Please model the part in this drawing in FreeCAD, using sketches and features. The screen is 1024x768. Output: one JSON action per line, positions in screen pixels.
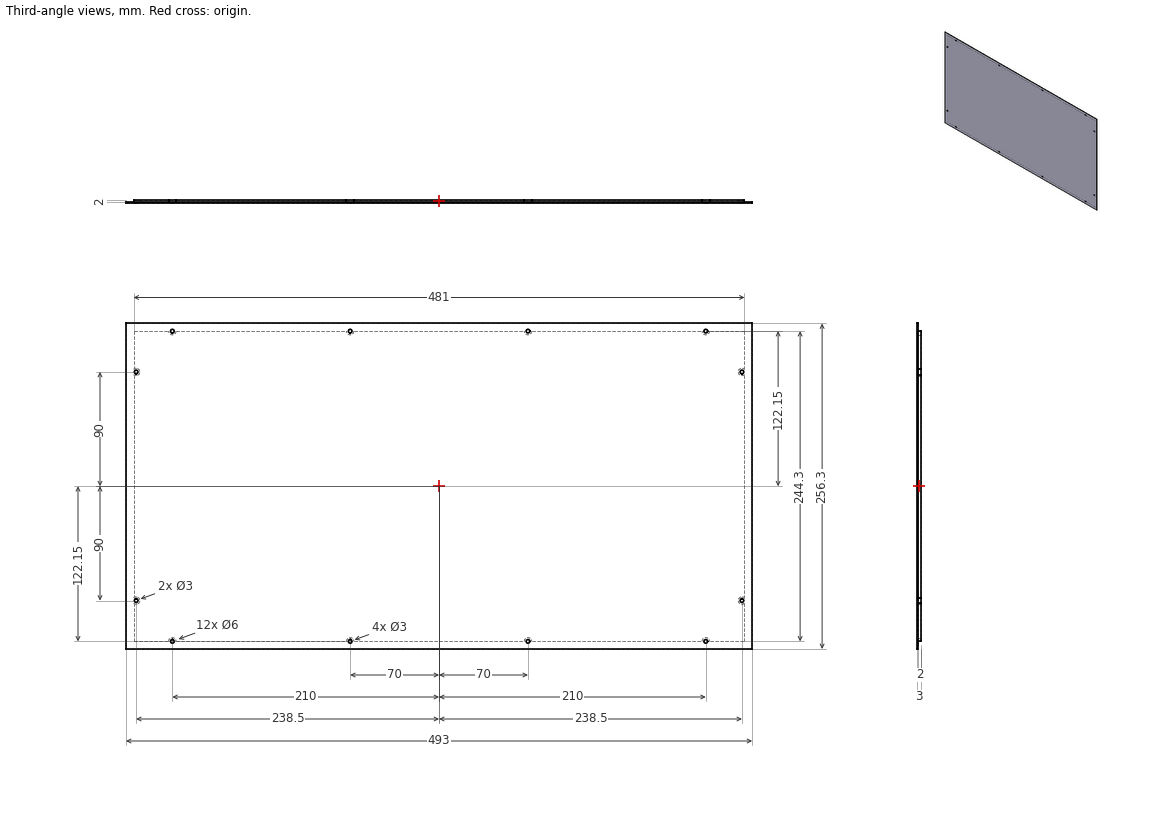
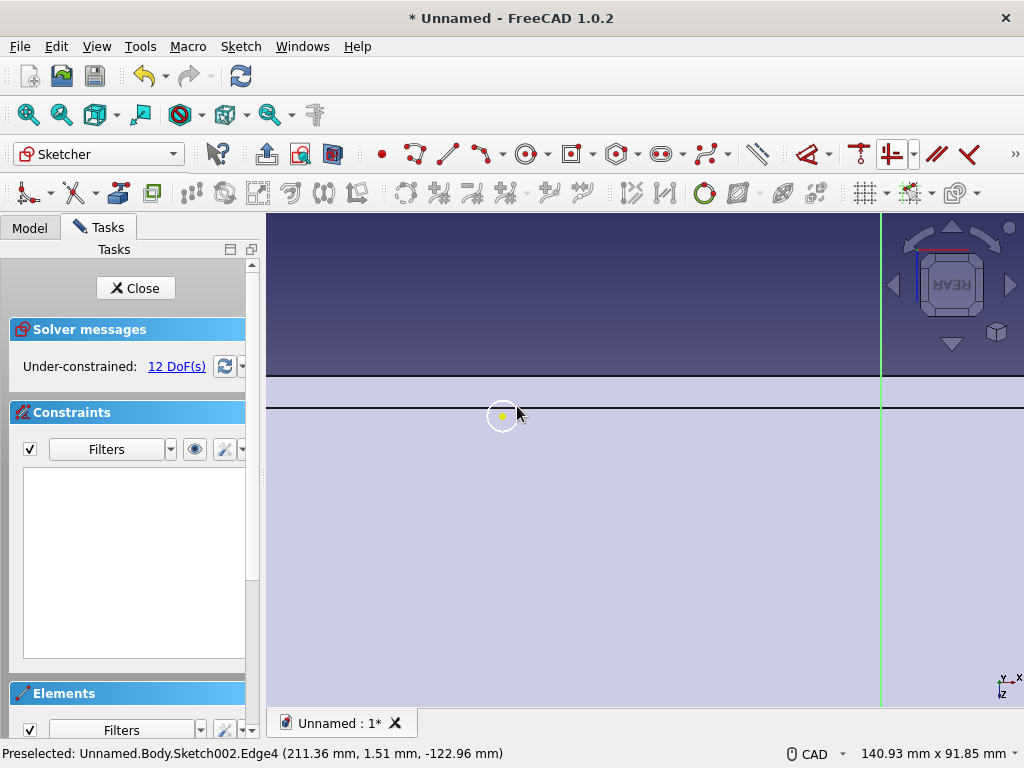
{"action": "left_click", "coordinate": [514, 405]}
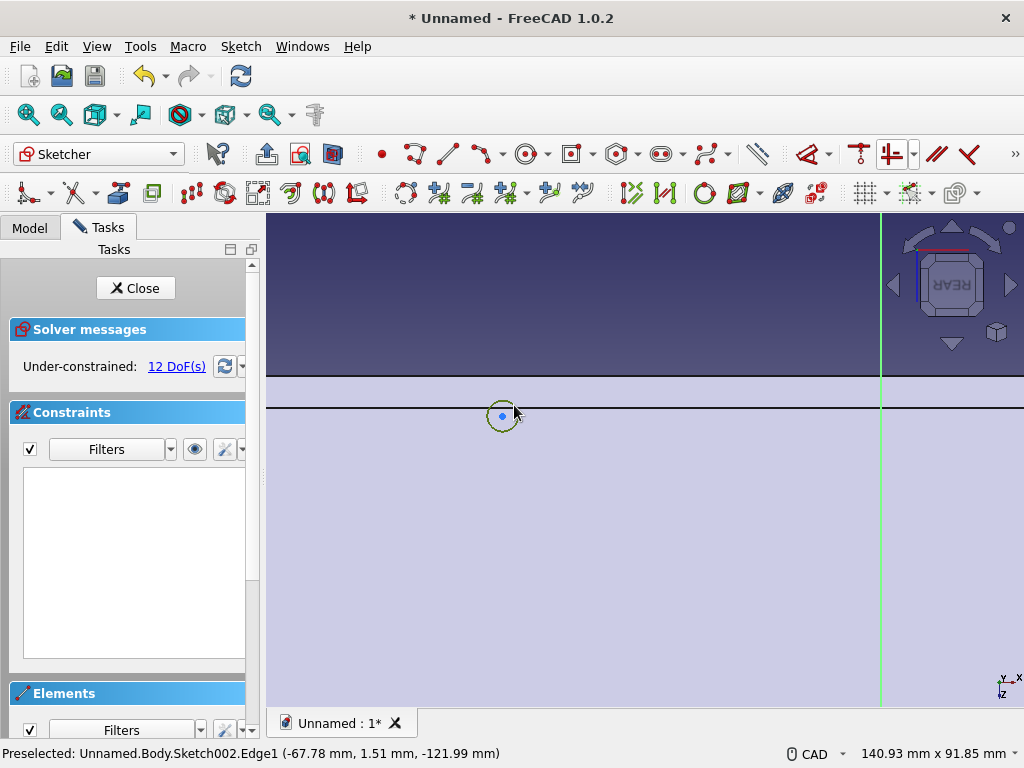
{"action": "scroll", "coordinate": [516, 406], "scroll_direction": "down", "scroll_amount": 9}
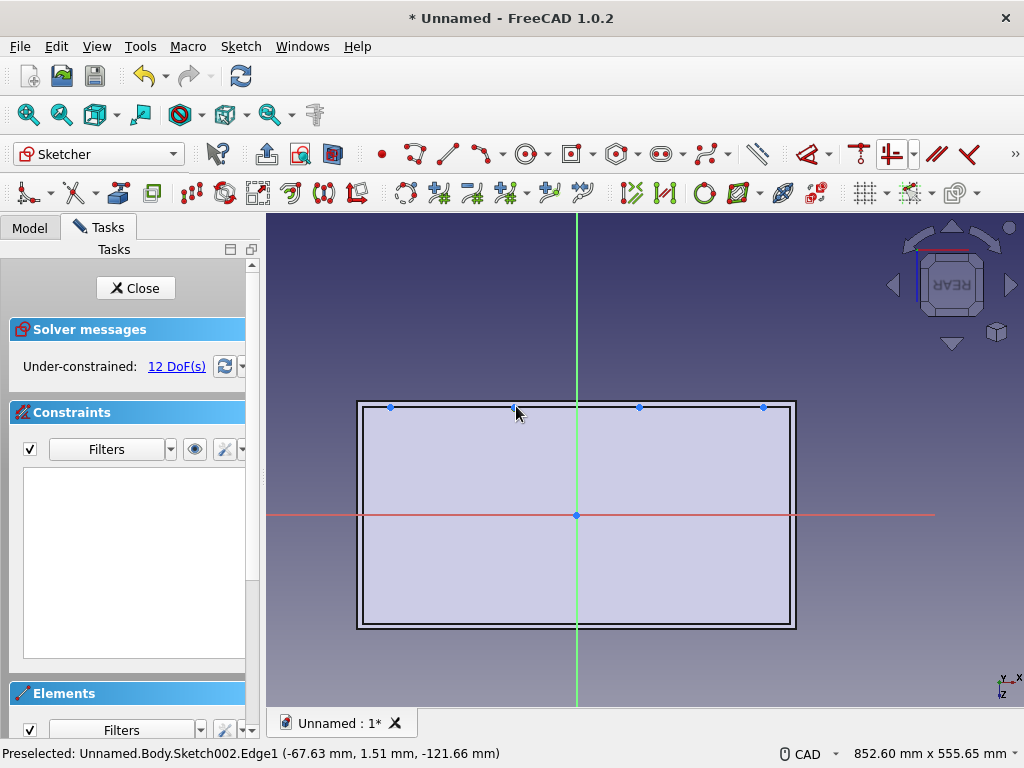
{"action": "scroll", "coordinate": [392, 406], "scroll_direction": "up", "scroll_amount": 9}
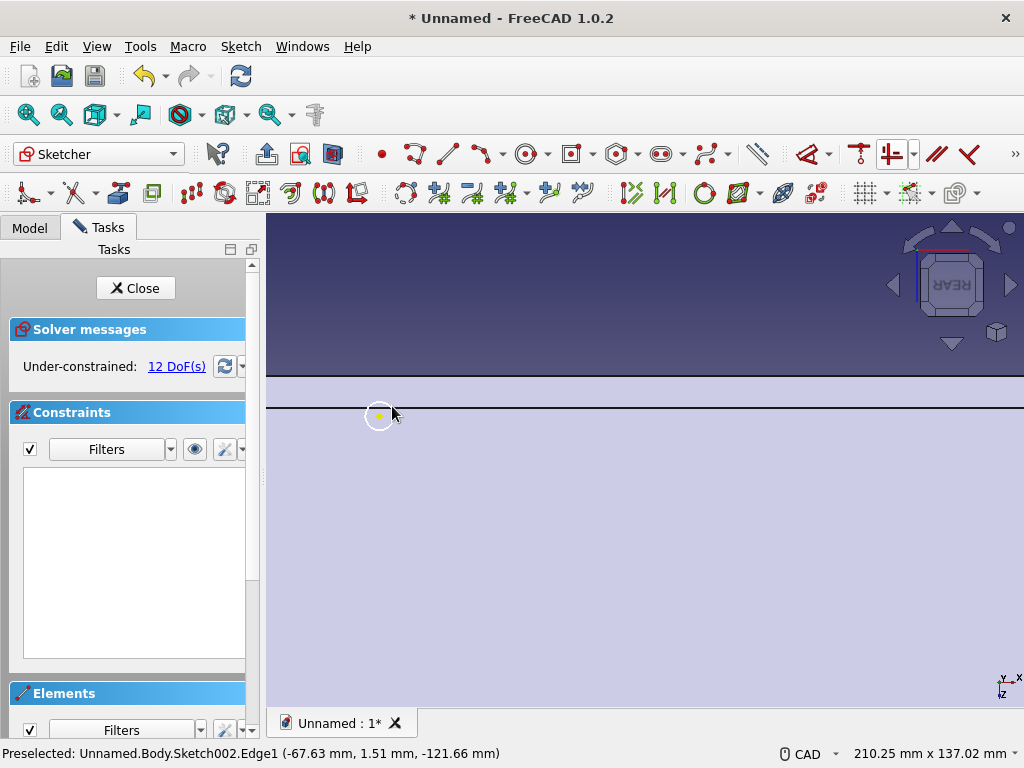
{"action": "left_click", "coordinate": [390, 406]}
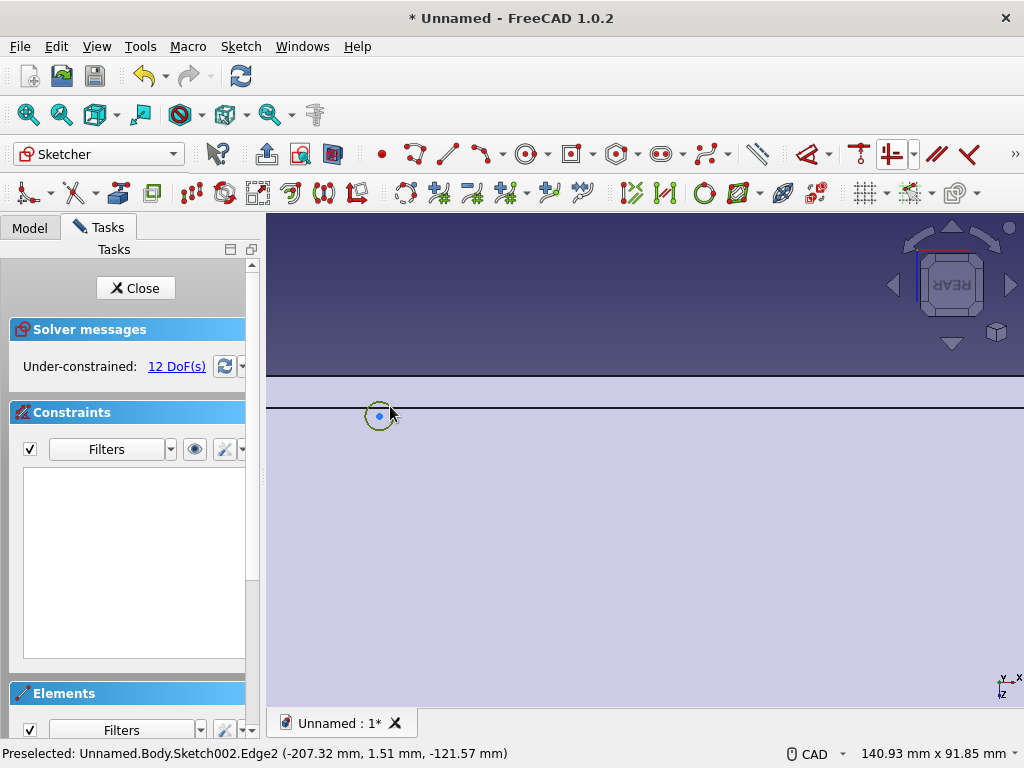
{"action": "scroll", "coordinate": [392, 406], "scroll_direction": "down", "scroll_amount": 9}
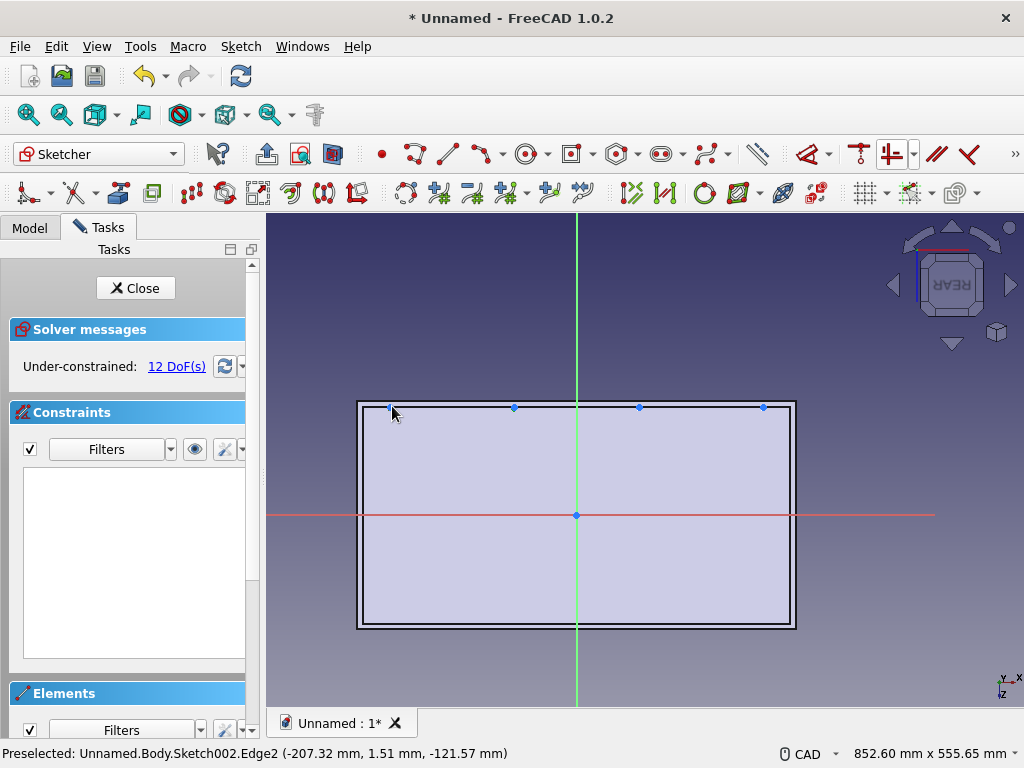
{"action": "scroll", "coordinate": [641, 406], "scroll_direction": "up", "scroll_amount": 9}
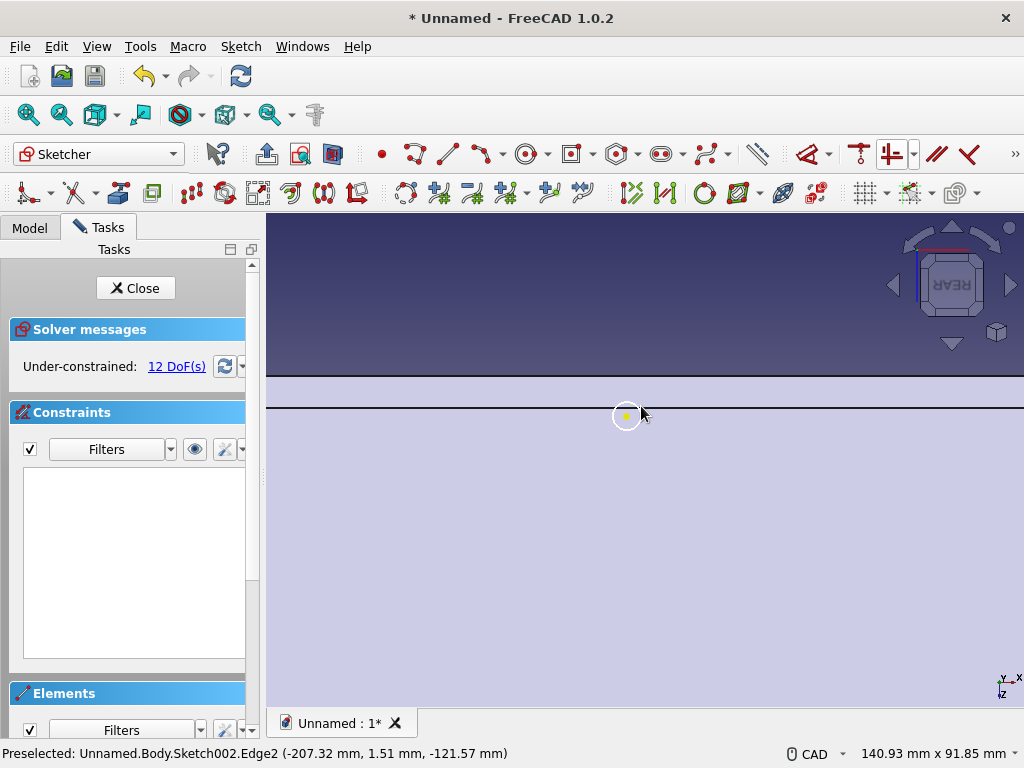
{"action": "left_click", "coordinate": [637, 406]}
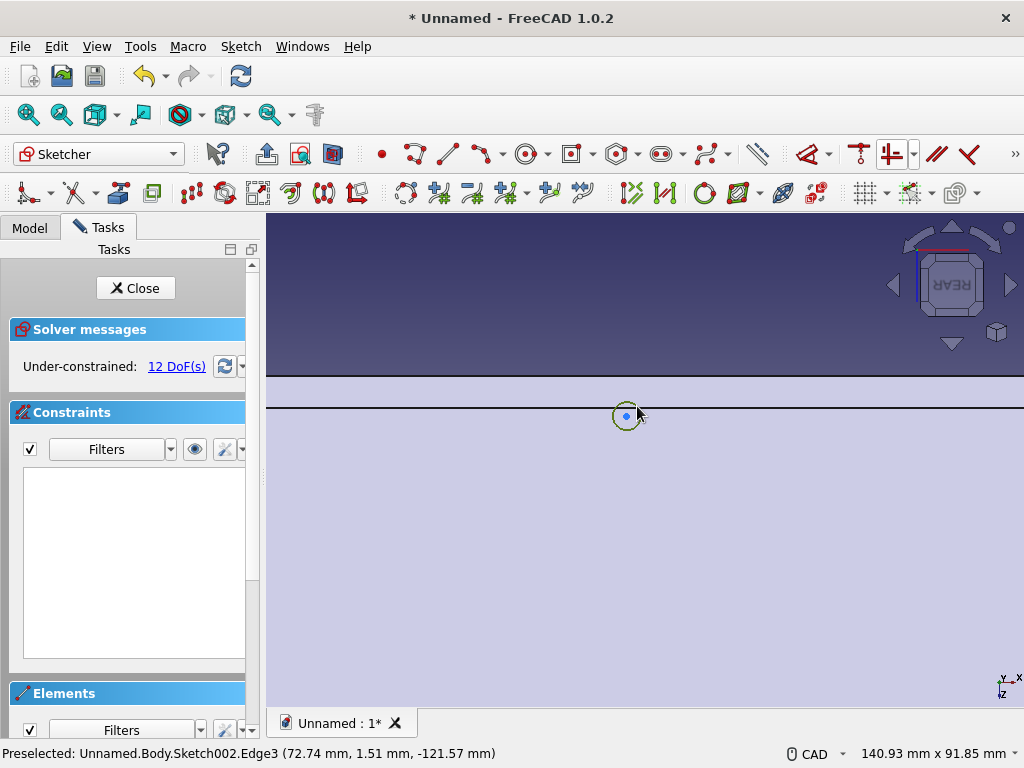
{"action": "scroll", "coordinate": [641, 406], "scroll_direction": "down", "scroll_amount": 9}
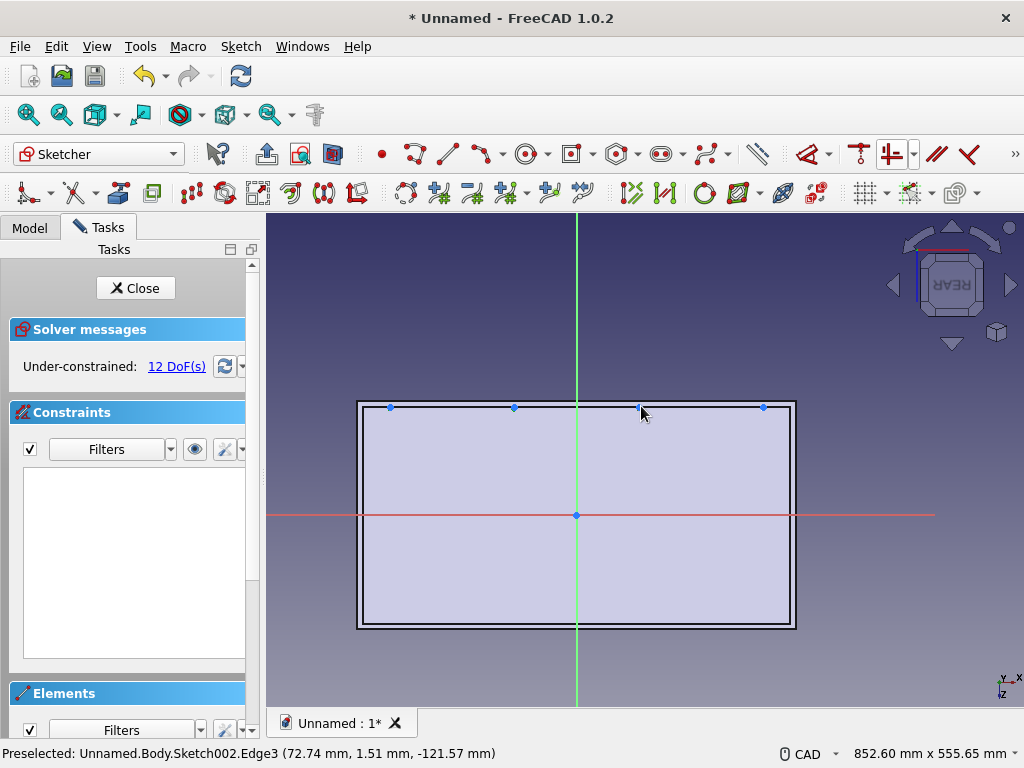
{"action": "scroll", "coordinate": [765, 406], "scroll_direction": "up", "scroll_amount": 9}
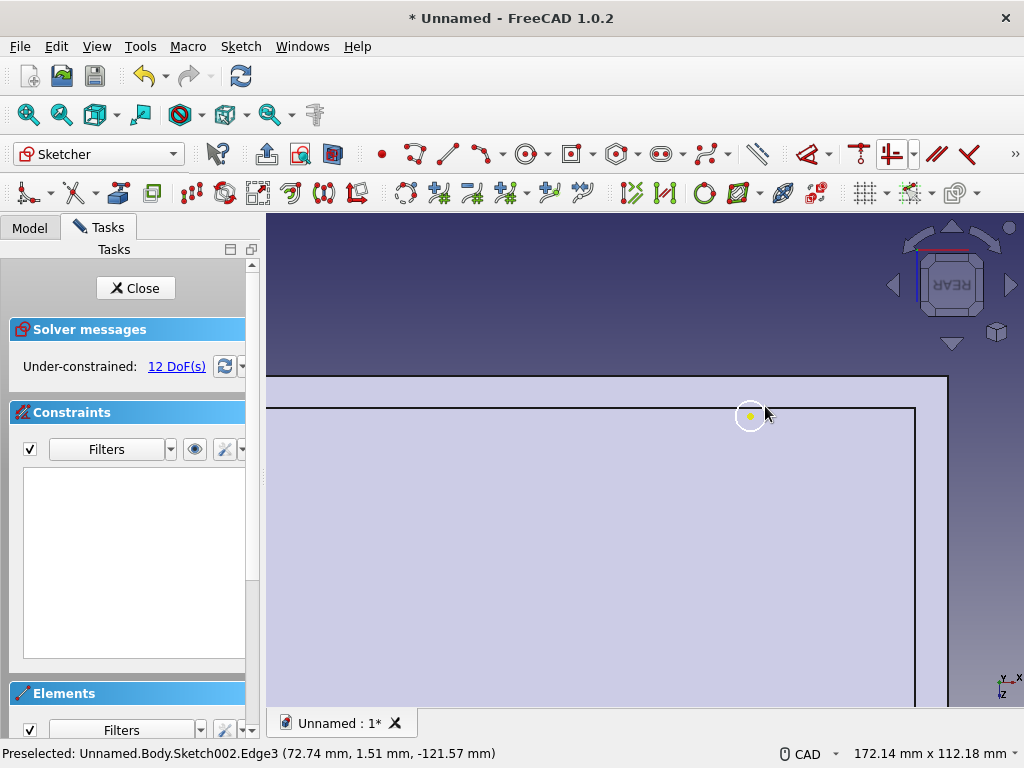
{"action": "left_click", "coordinate": [761, 405]}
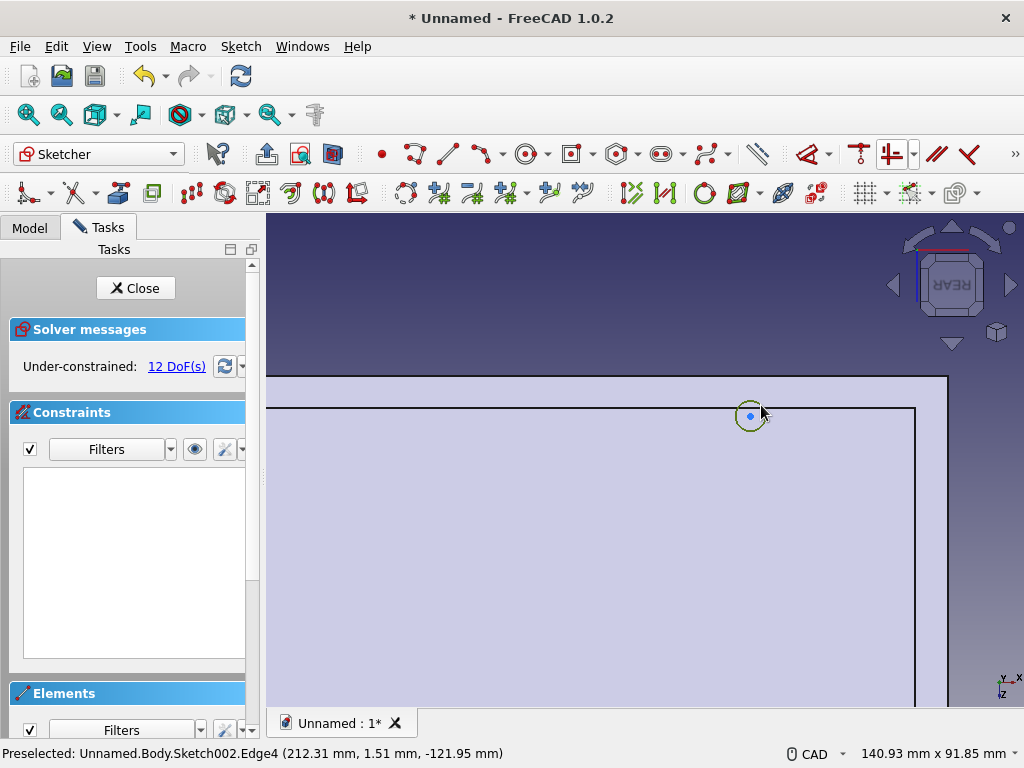
{"action": "key", "text": "e"}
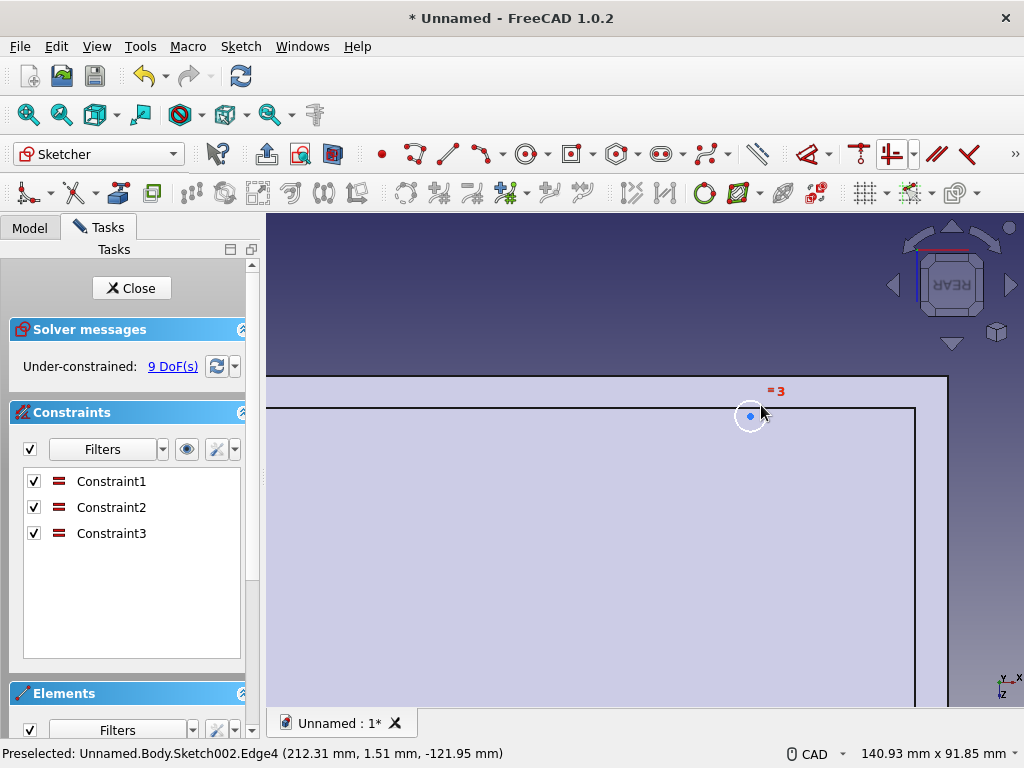
{"action": "scroll", "coordinate": [766, 406], "scroll_direction": "down", "scroll_amount": 9}